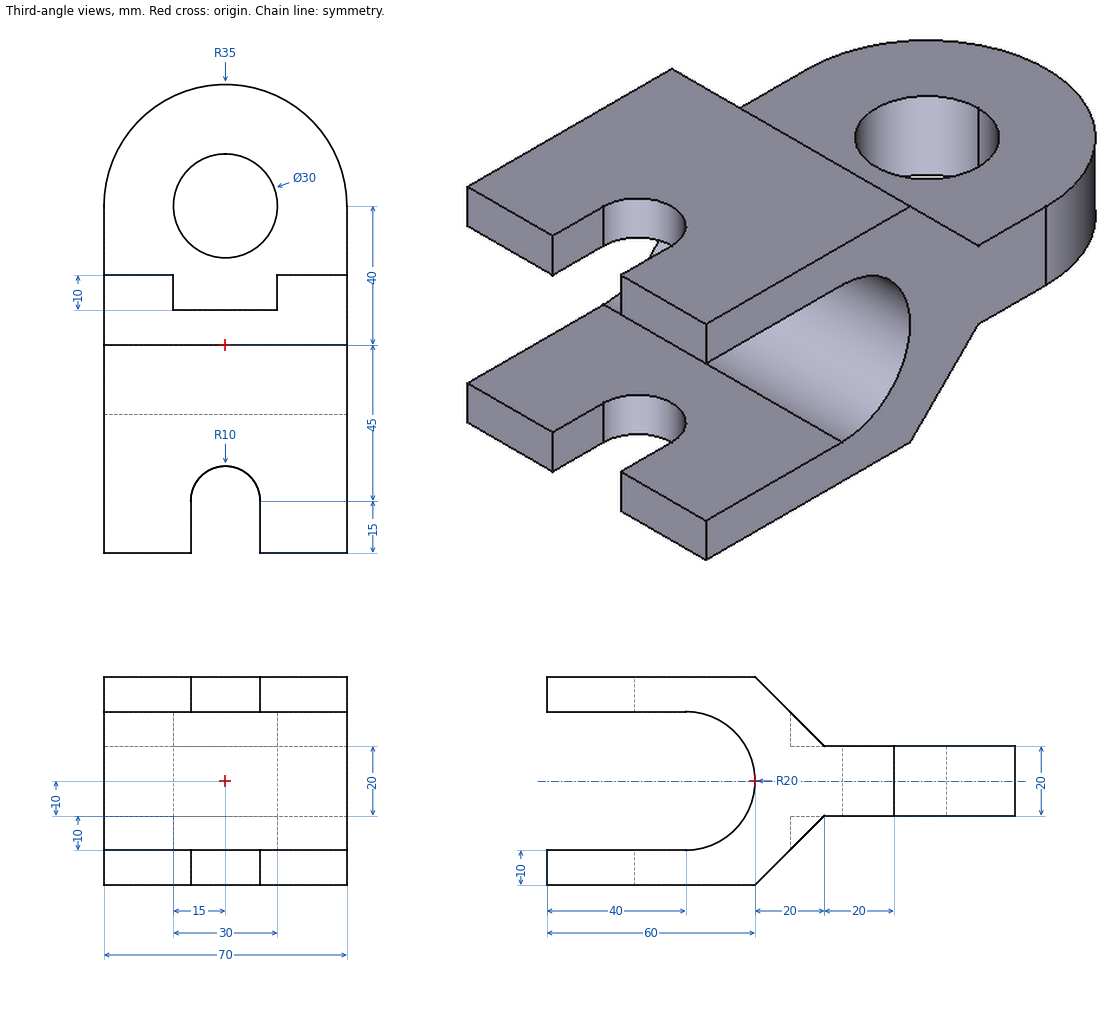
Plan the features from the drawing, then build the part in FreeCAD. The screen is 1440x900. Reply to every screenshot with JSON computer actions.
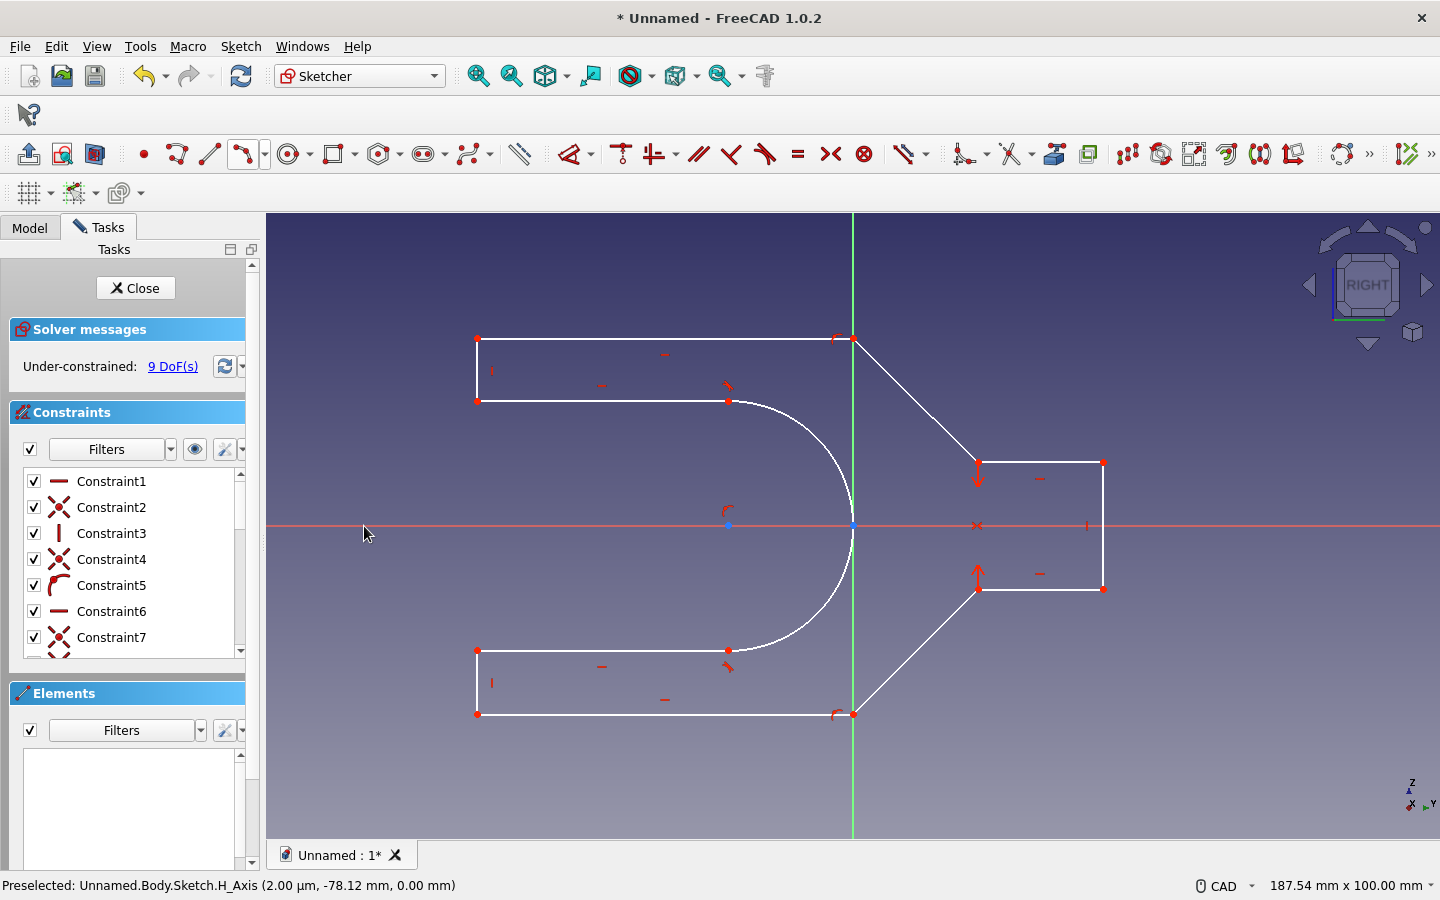
{"action": "left_click", "coordinate": [477, 715]}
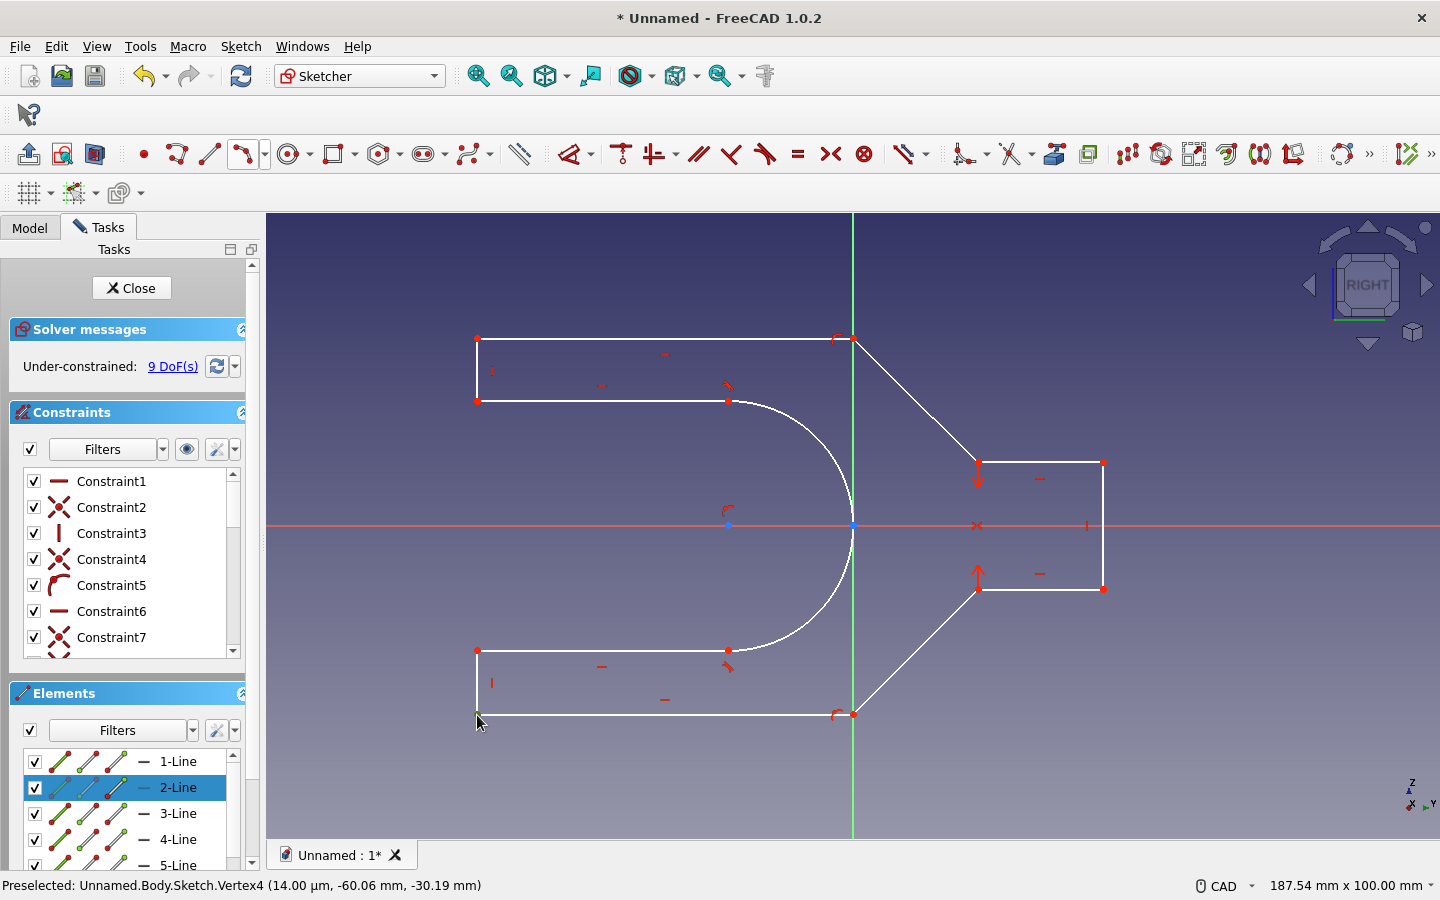
{"action": "left_click", "coordinate": [477, 339]}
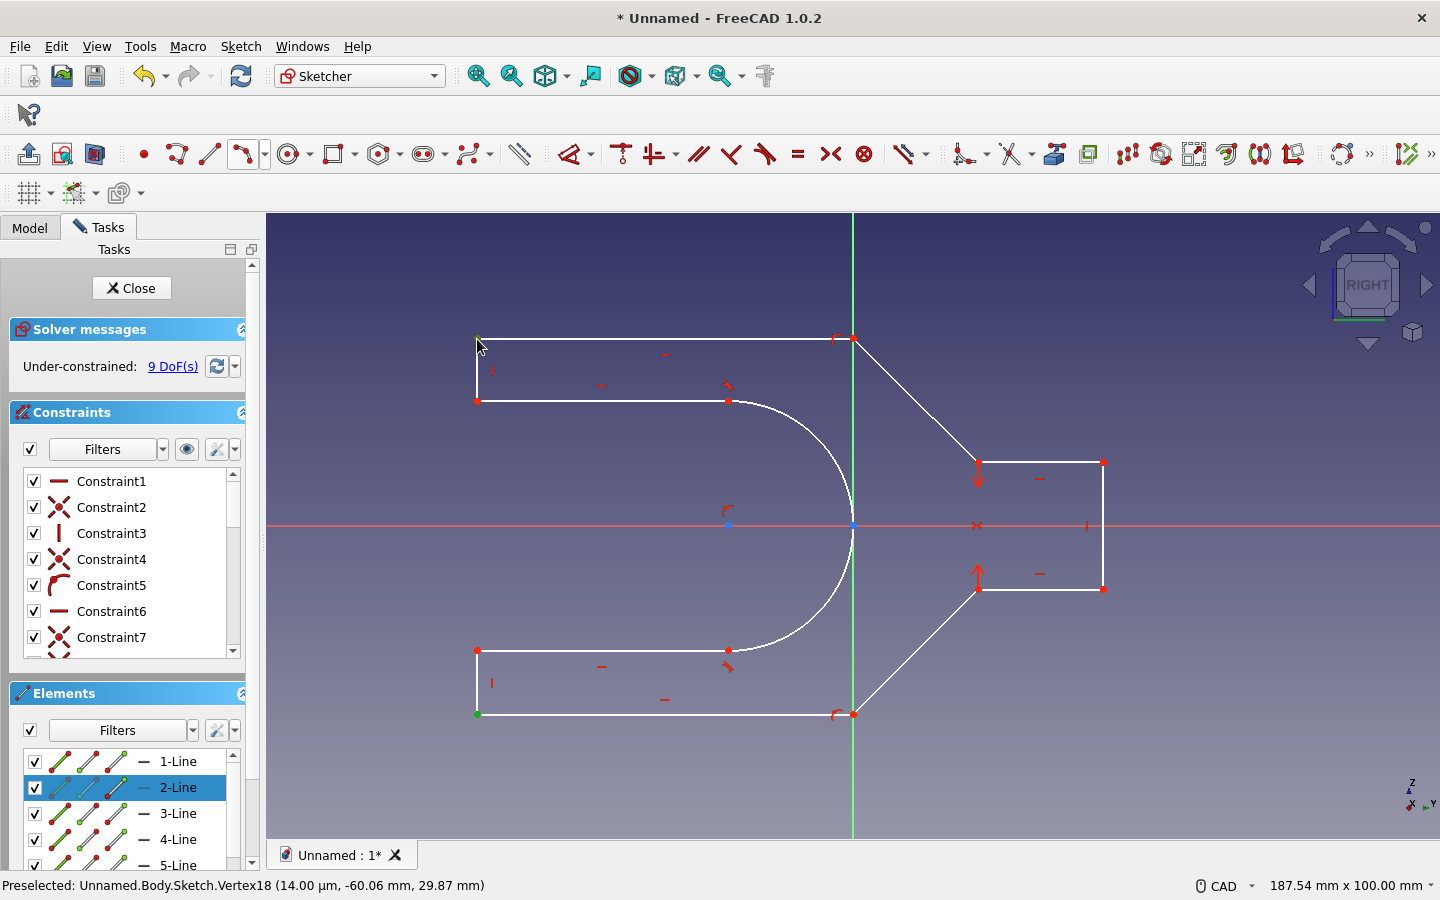
{"action": "left_click", "coordinate": [364, 526]}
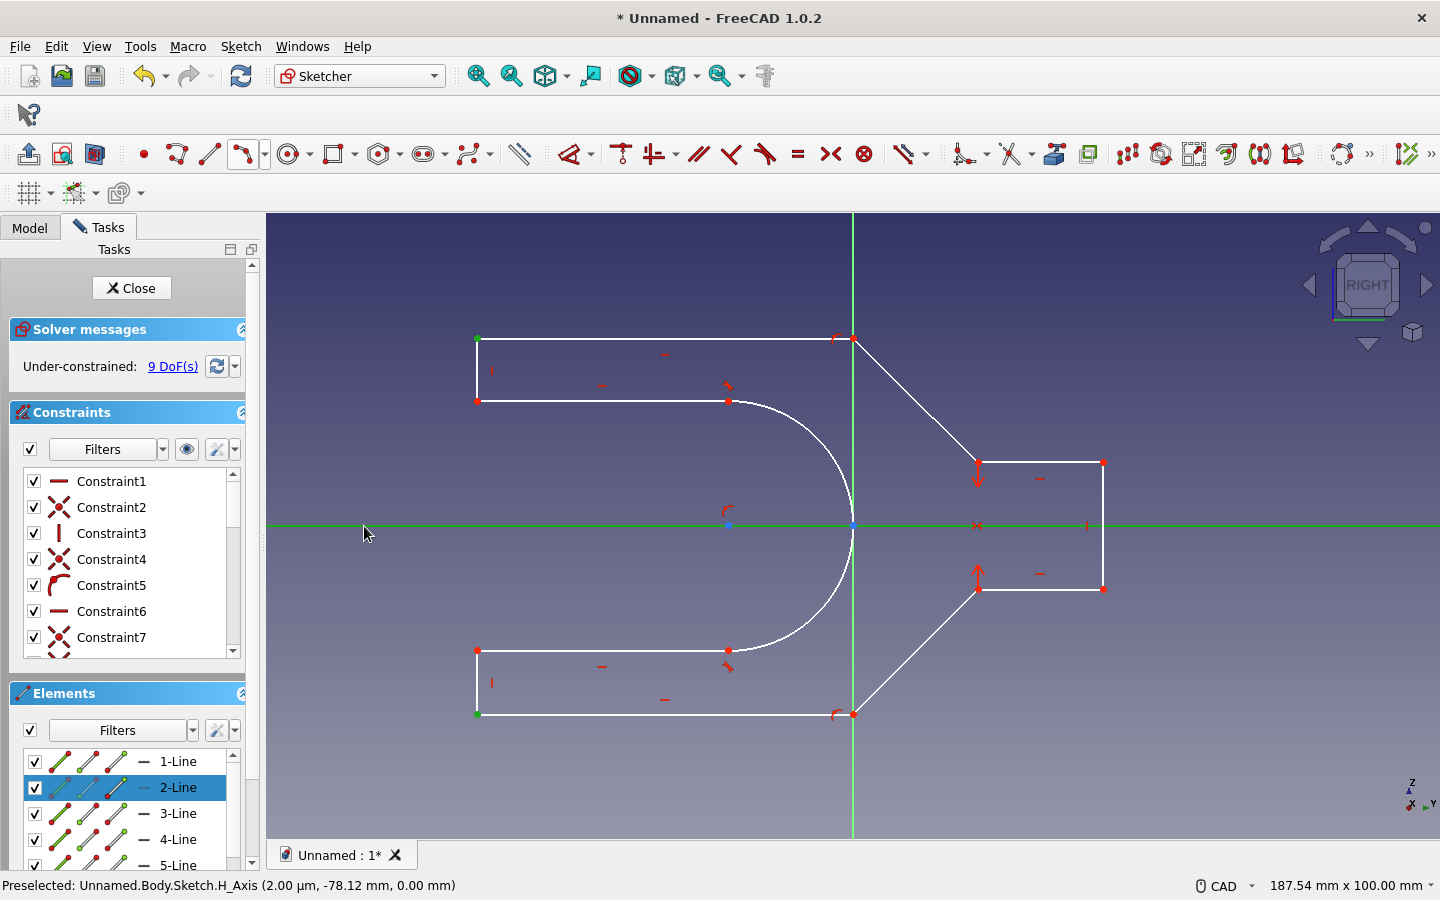
{"action": "key", "text": "s"}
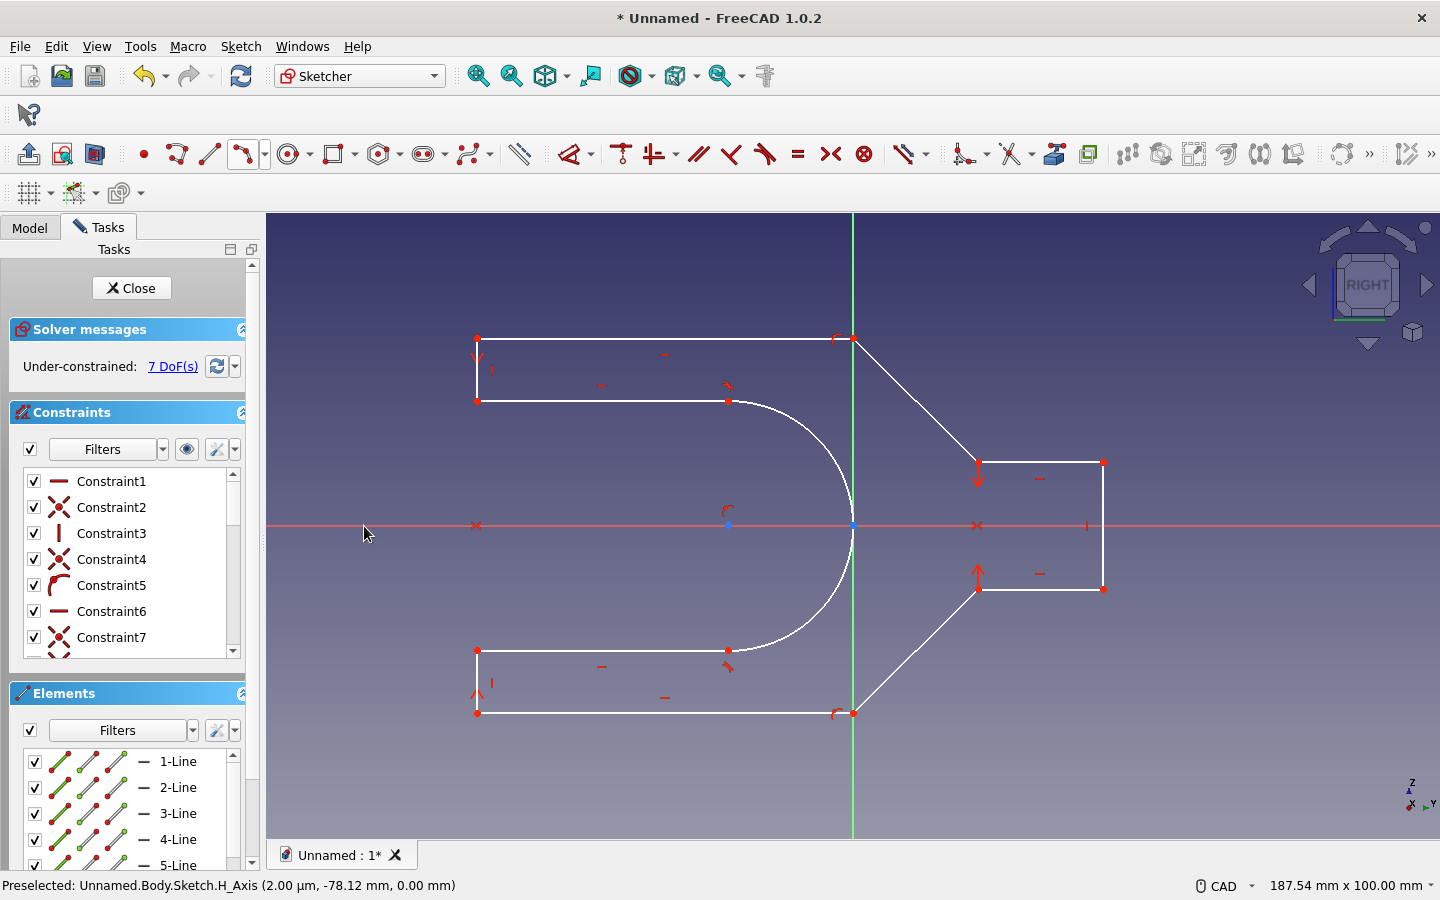
{"action": "key", "text": "d"}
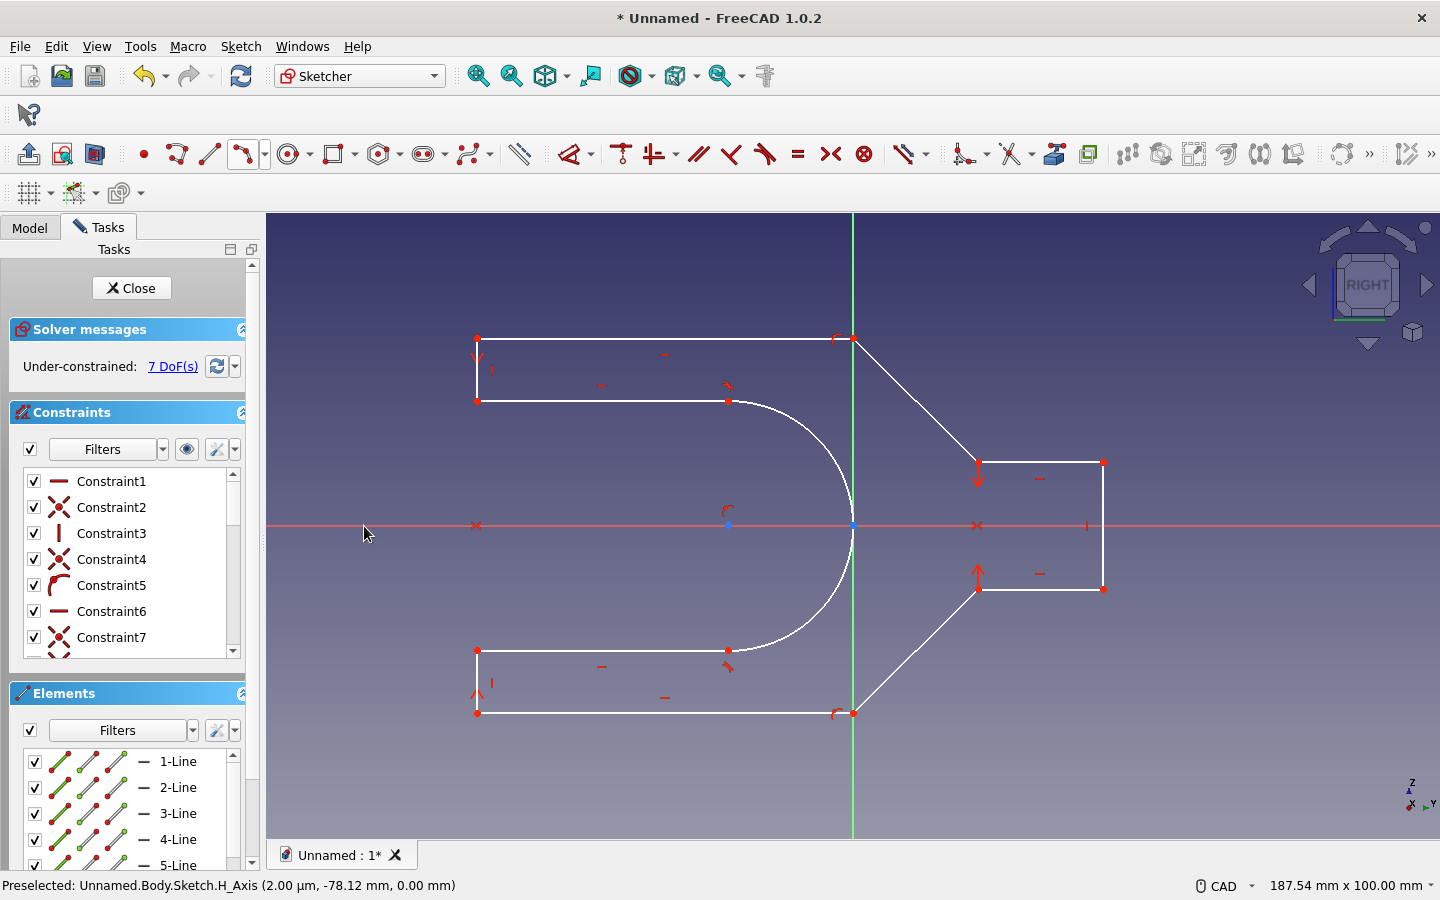
{"action": "left_click", "coordinate": [829, 599]}
{"action": "left_click", "coordinate": [795, 667]}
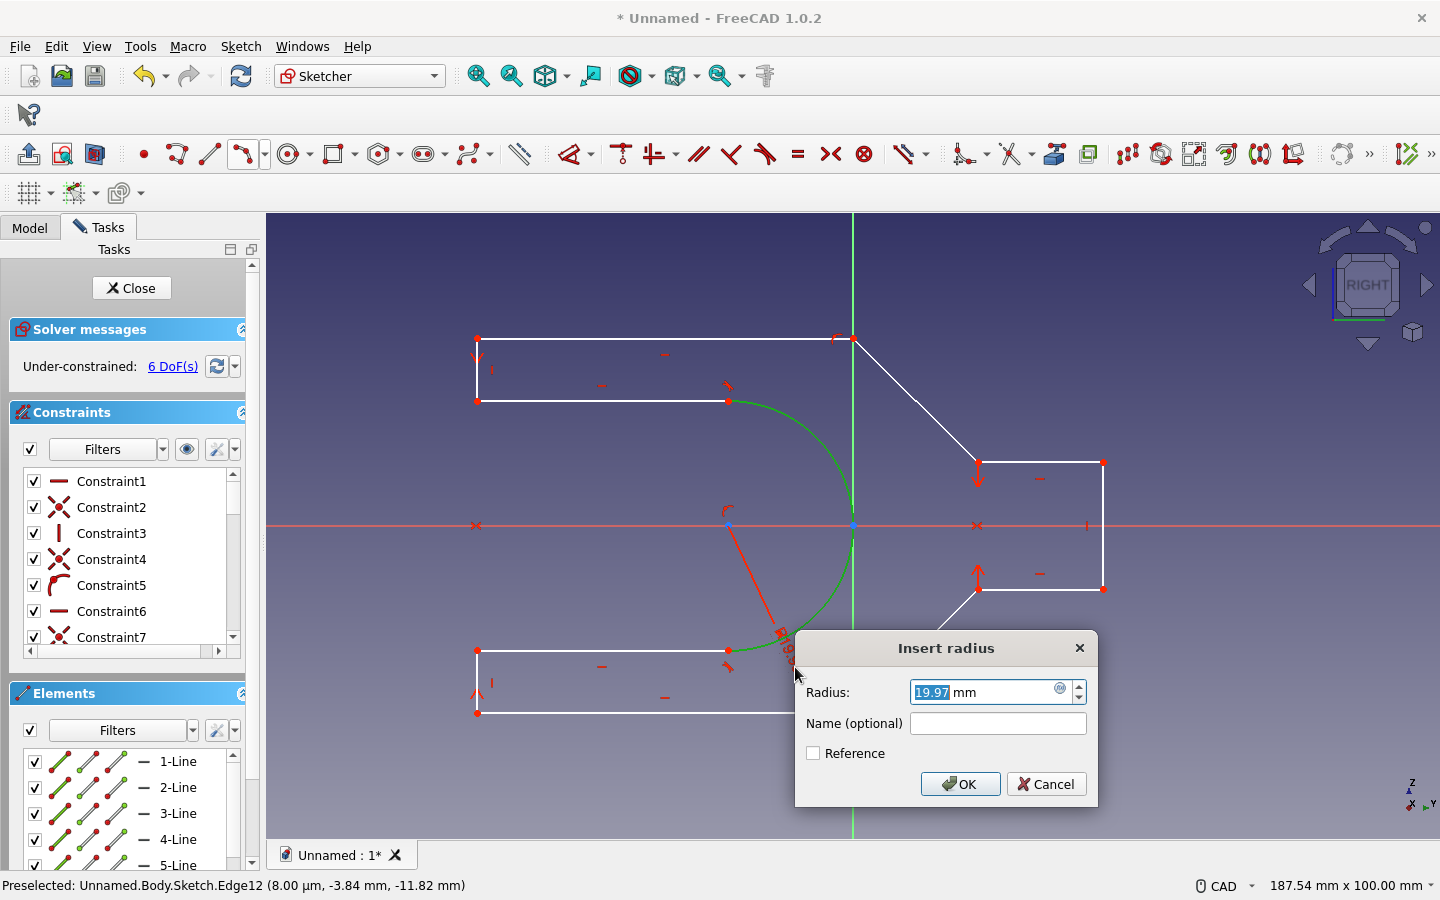
{"action": "type", "text": "20"}
{"action": "key", "text": "Return"}